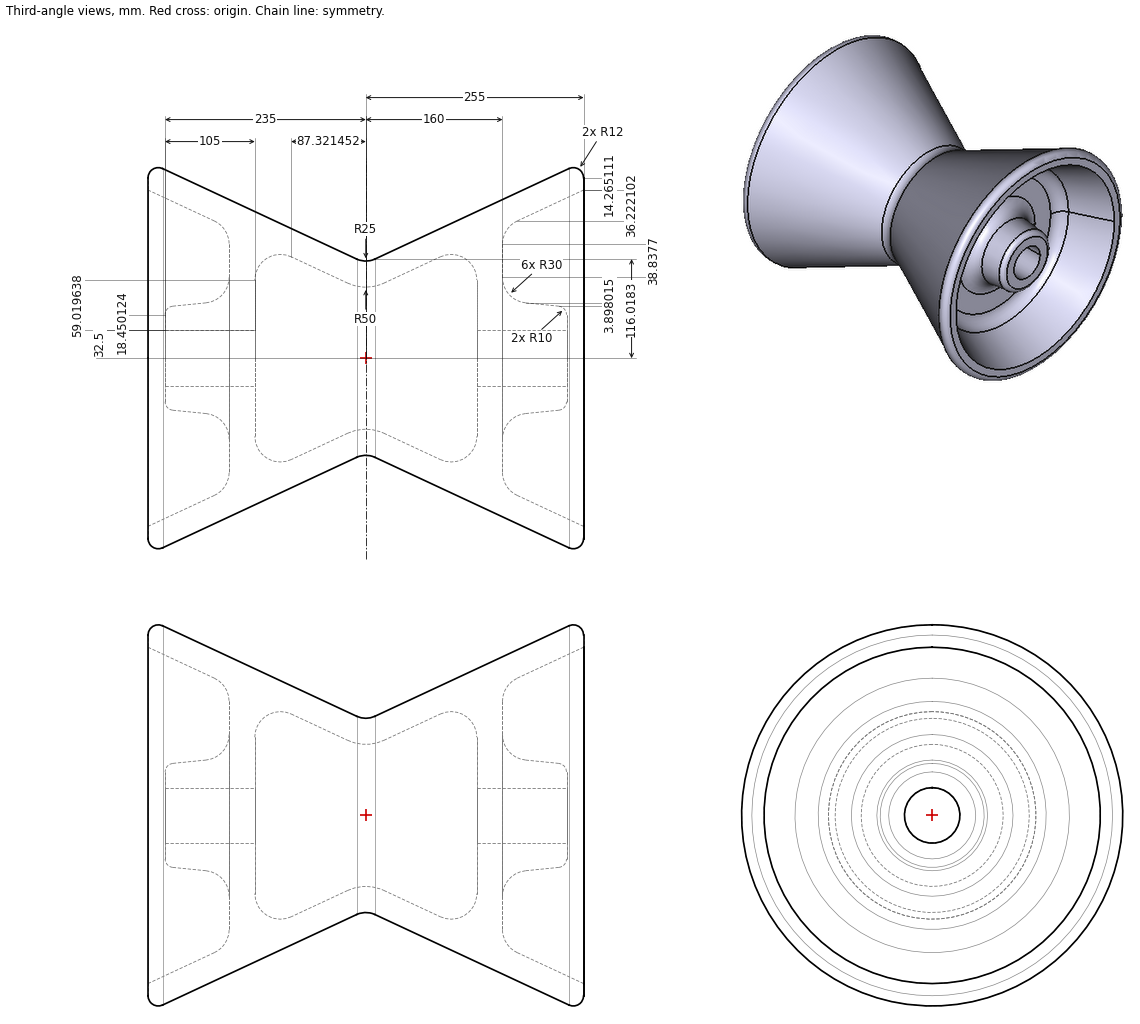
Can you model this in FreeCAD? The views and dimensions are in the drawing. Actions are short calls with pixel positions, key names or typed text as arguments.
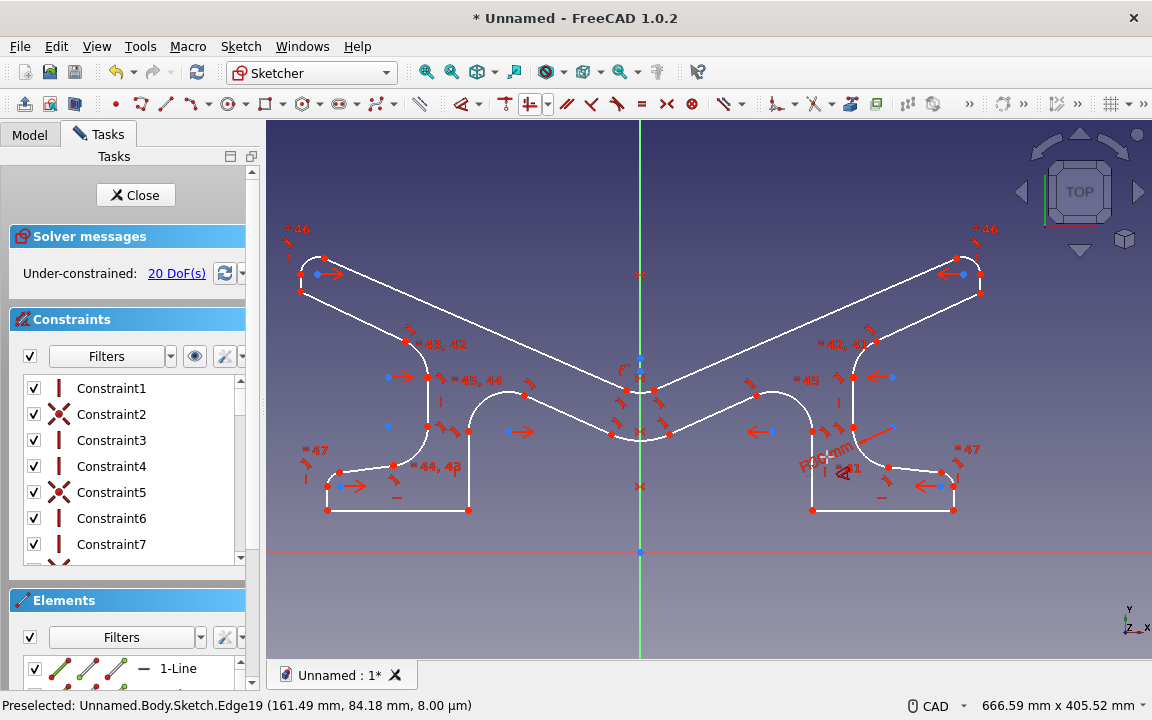
scroll(977, 265, up, 5)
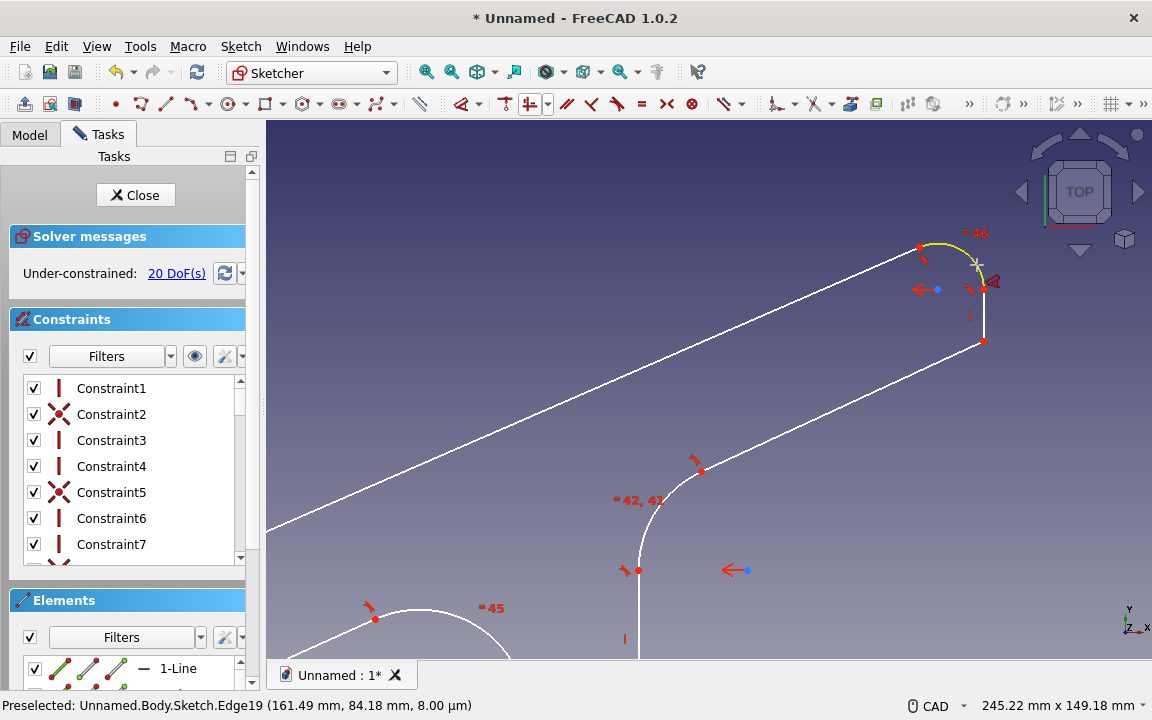
click(976, 264)
click(974, 220)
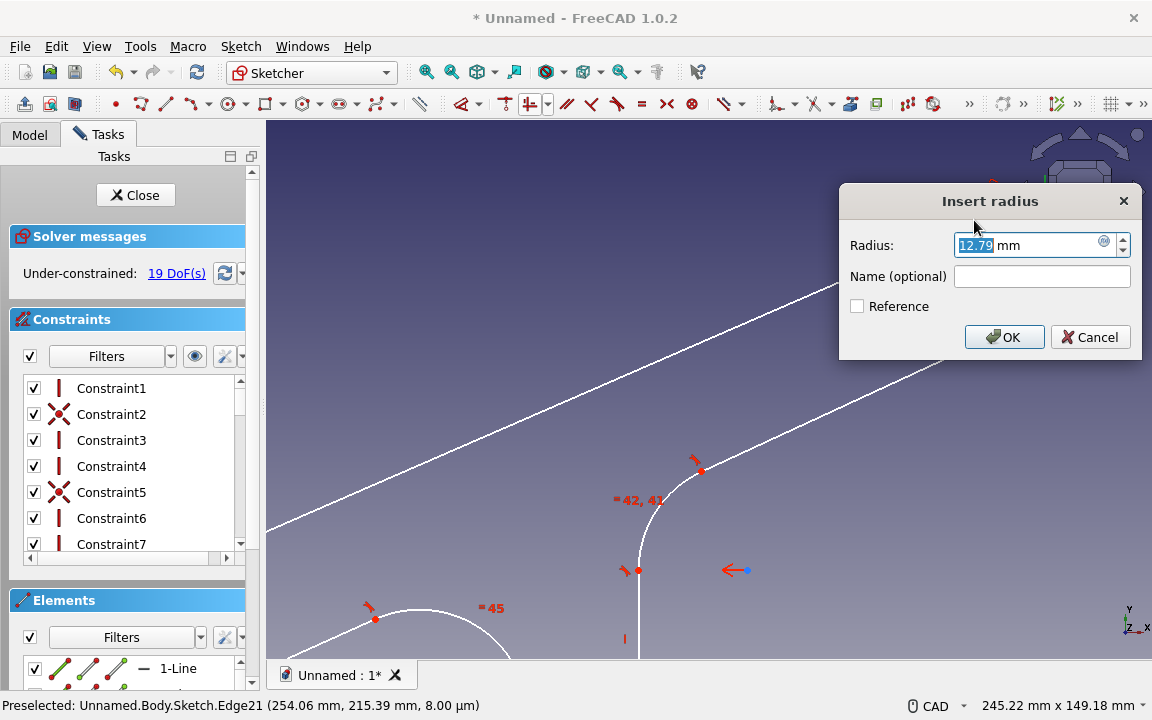
text(12)
key(Return)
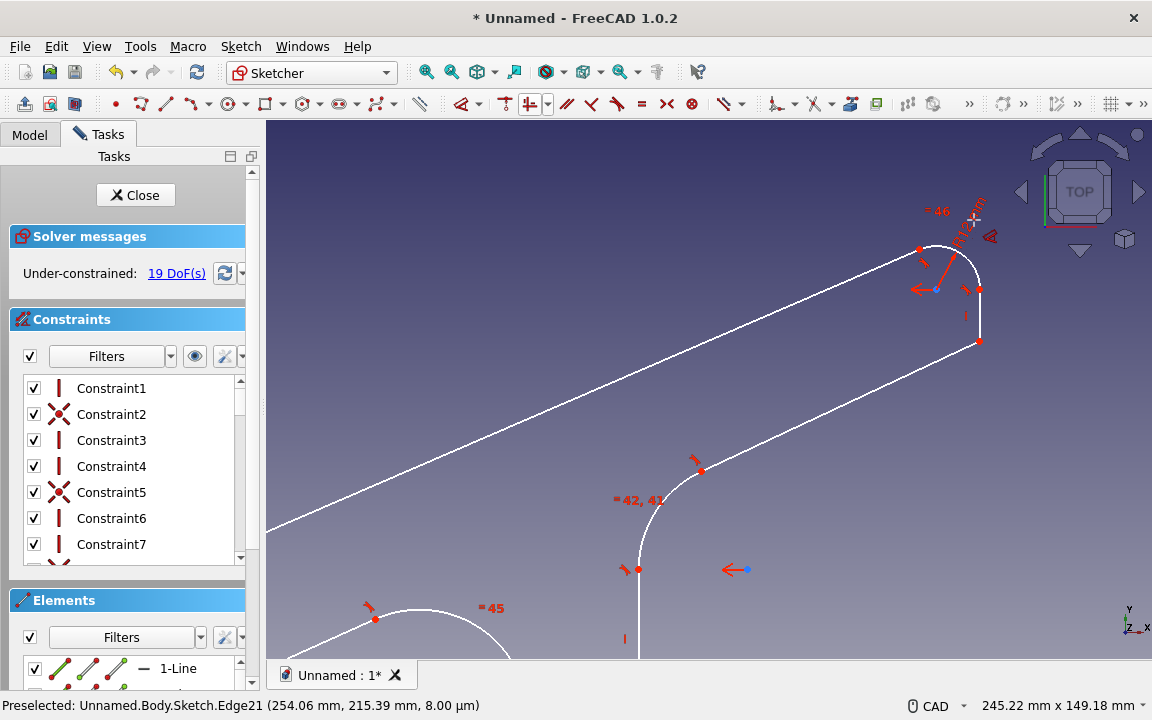
scroll(830, 306, down, 7)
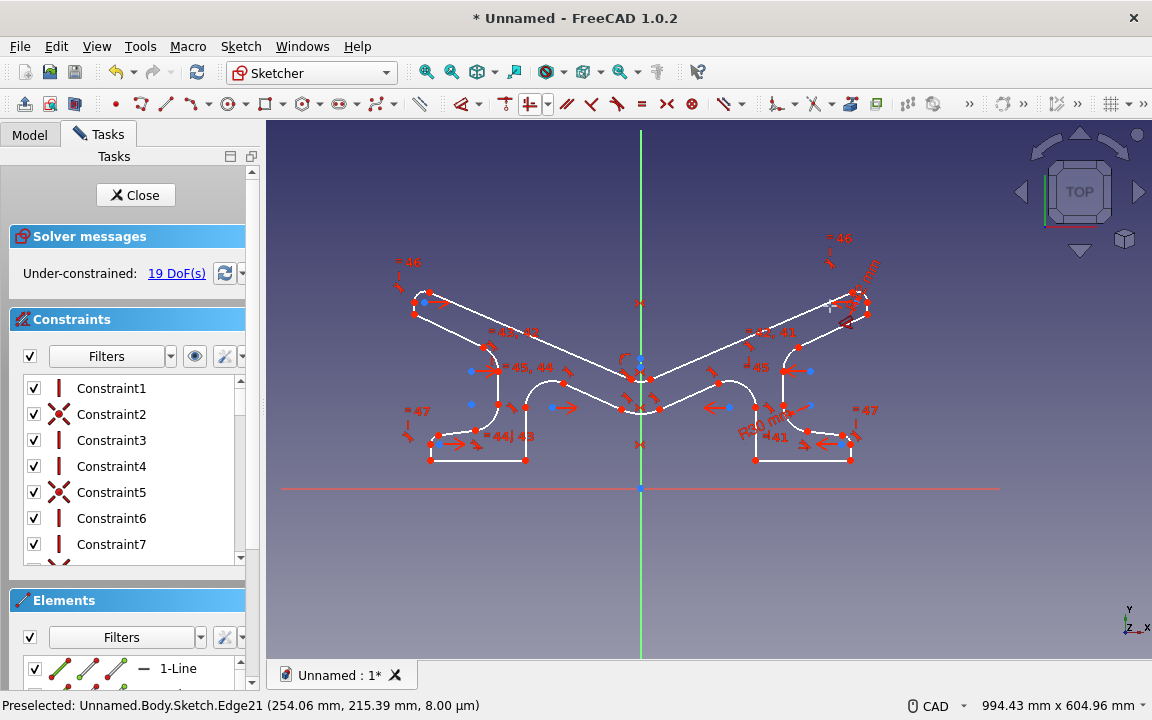
scroll(637, 382, up, 7)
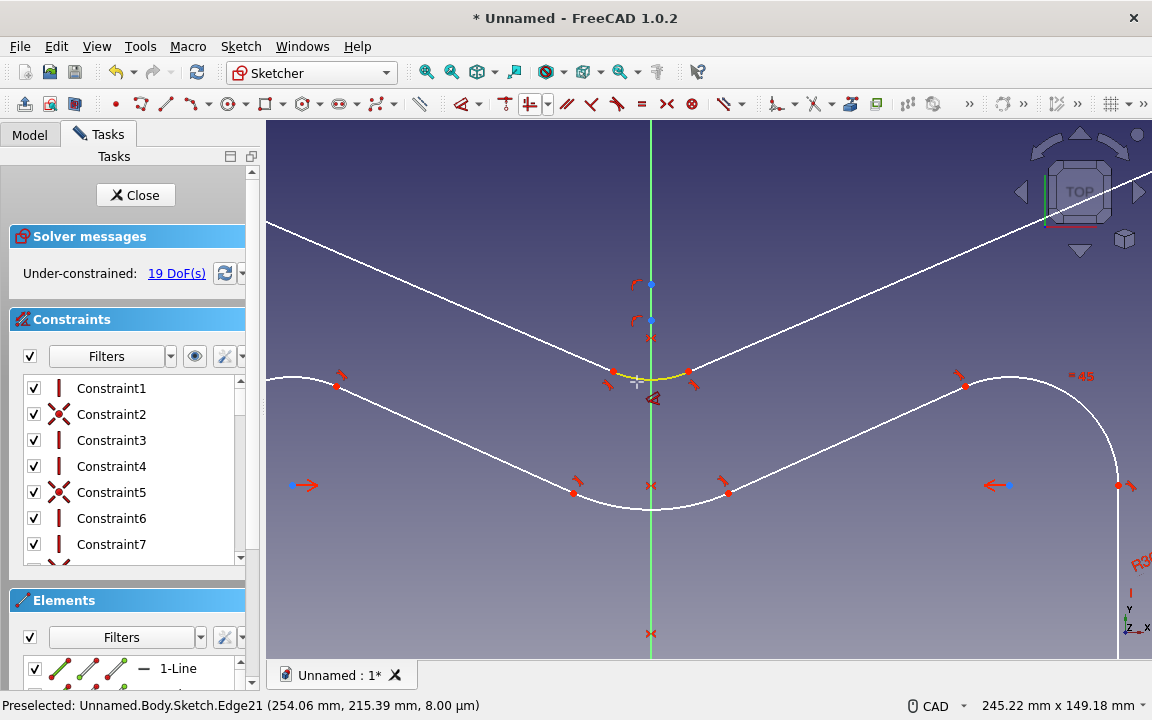
click(636, 379)
click(631, 411)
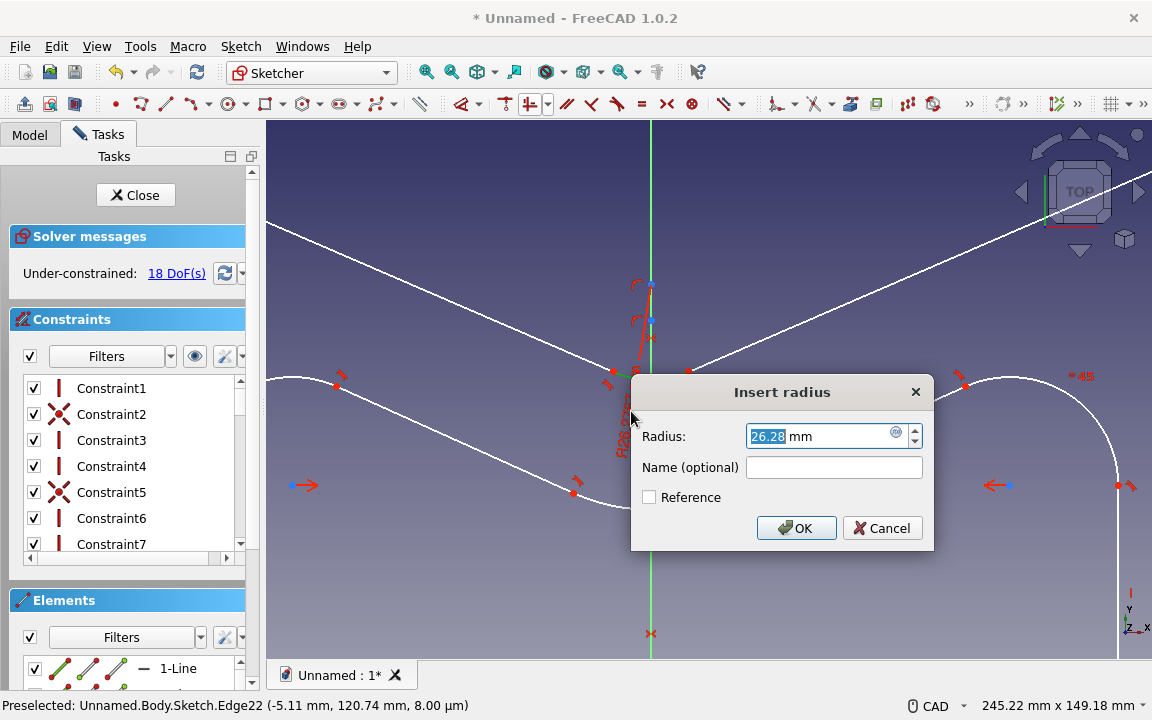
text(25)
key(Return)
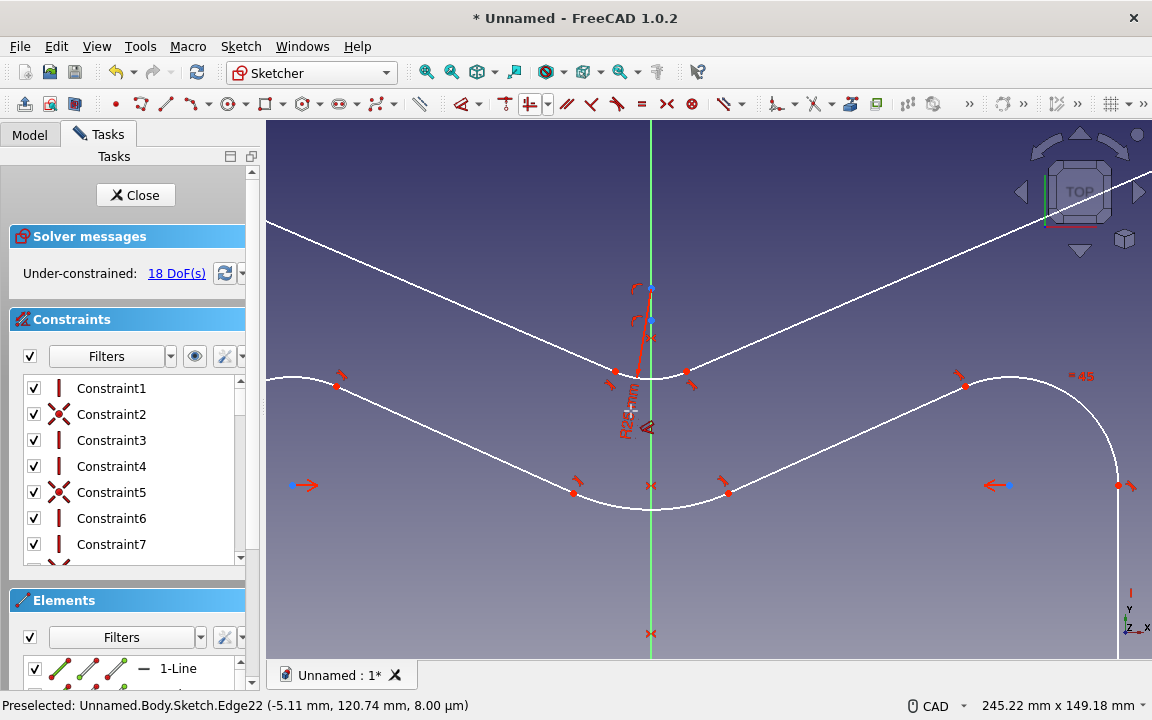
scroll(637, 382, down, 7)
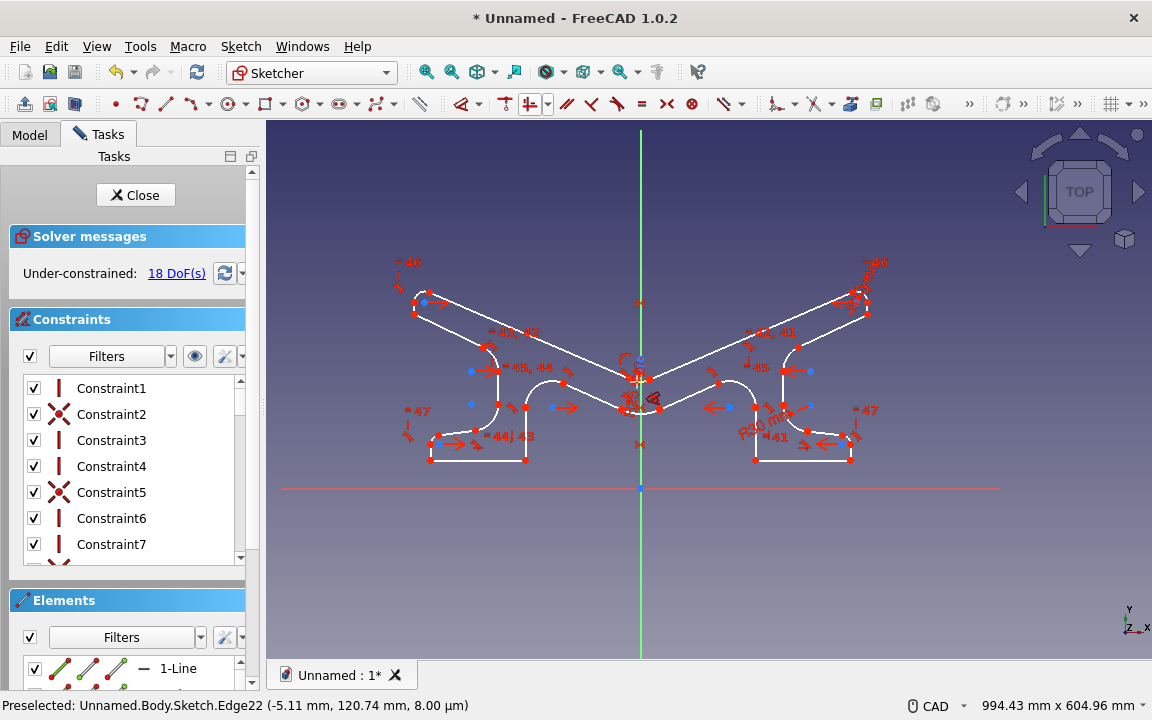
scroll(435, 437, up, 8)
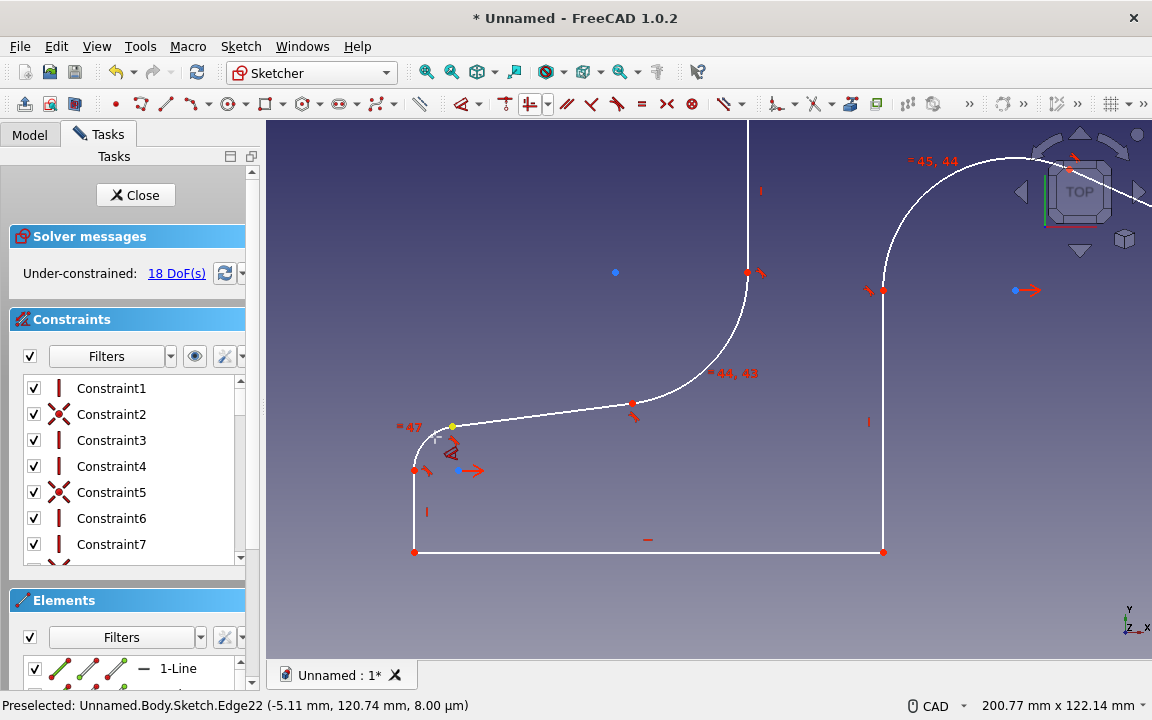
click(435, 433)
click(418, 406)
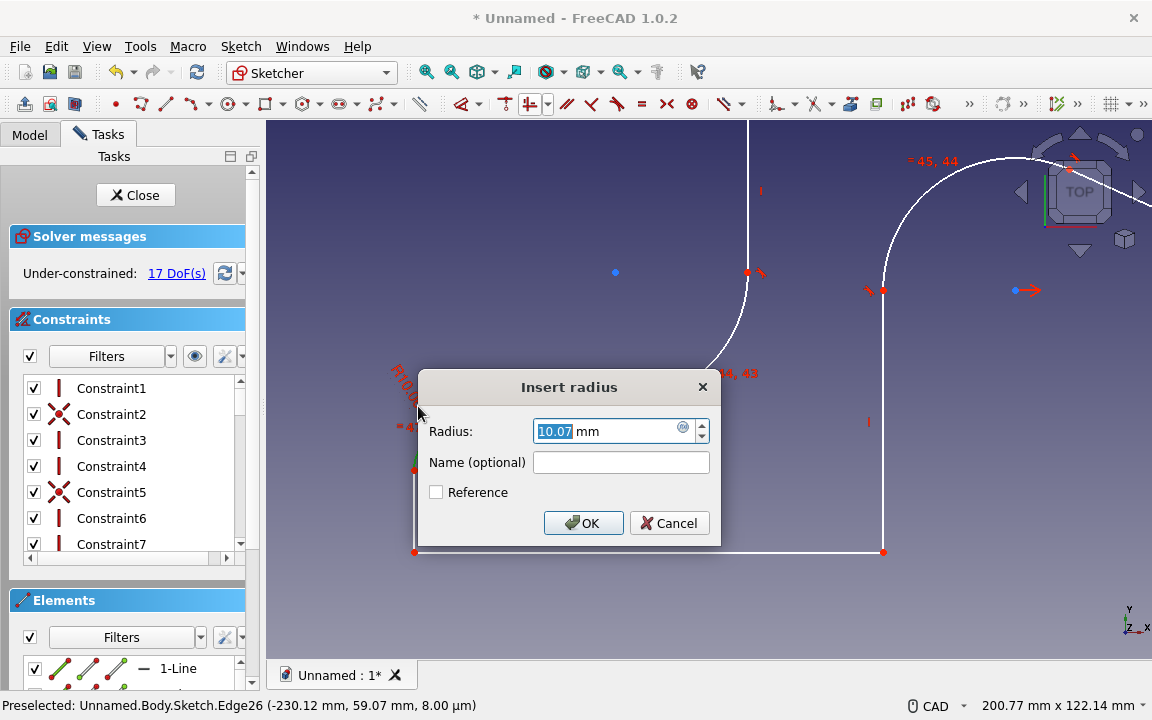
text(10)
key(Return)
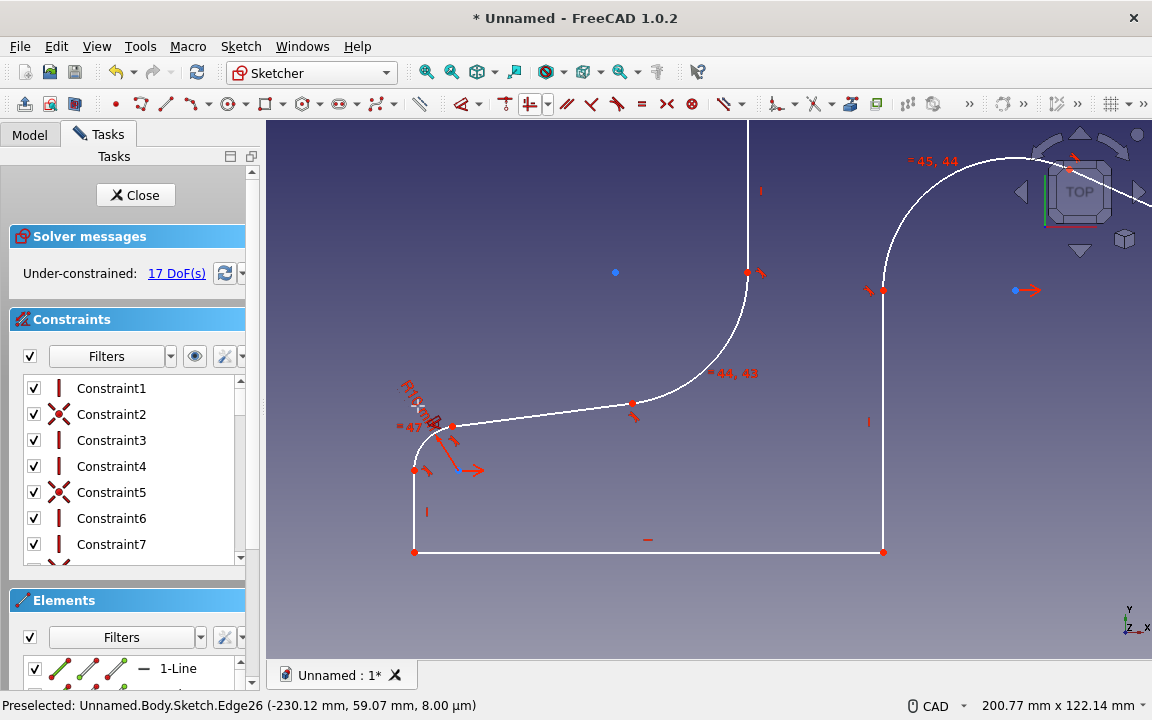
scroll(435, 437, down, 8)